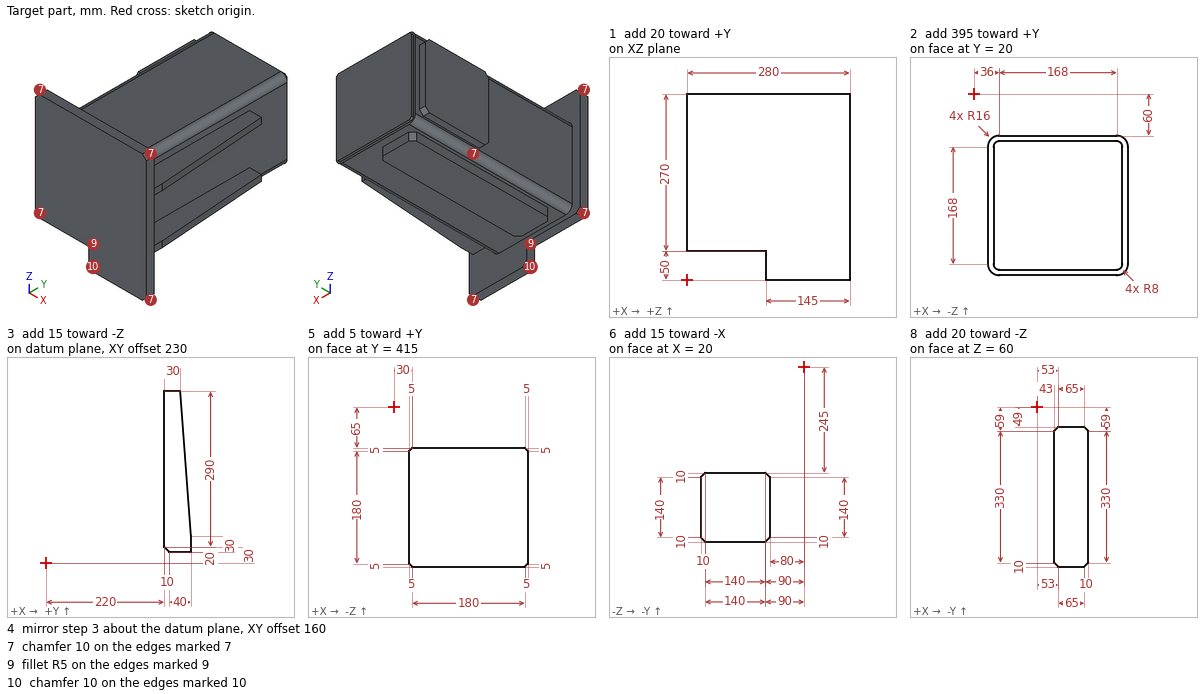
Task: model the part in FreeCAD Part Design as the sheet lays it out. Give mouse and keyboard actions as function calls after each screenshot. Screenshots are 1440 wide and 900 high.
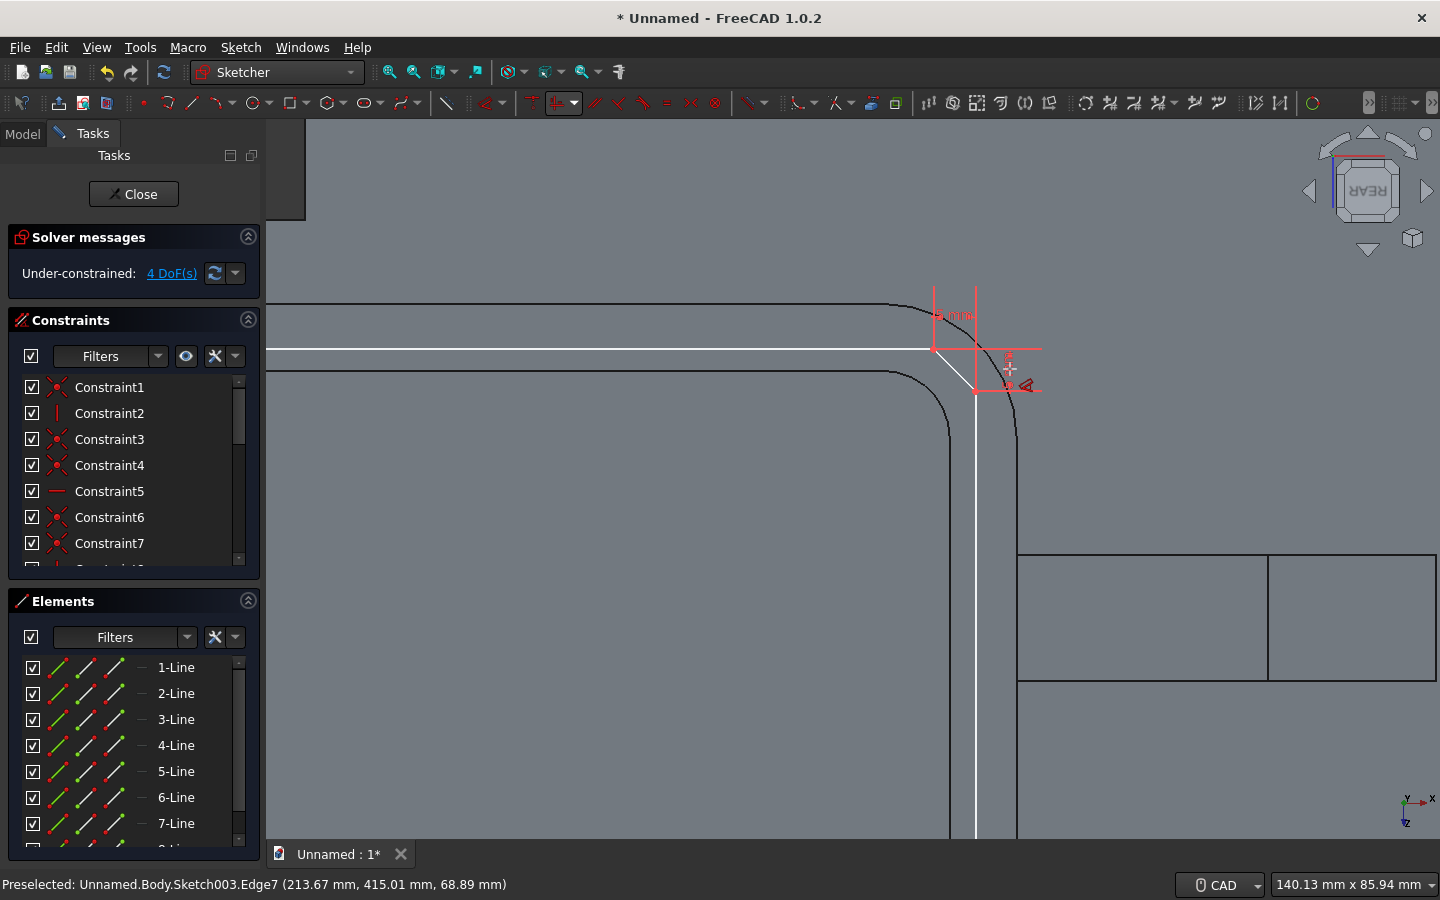
scroll(964, 380, down, 8)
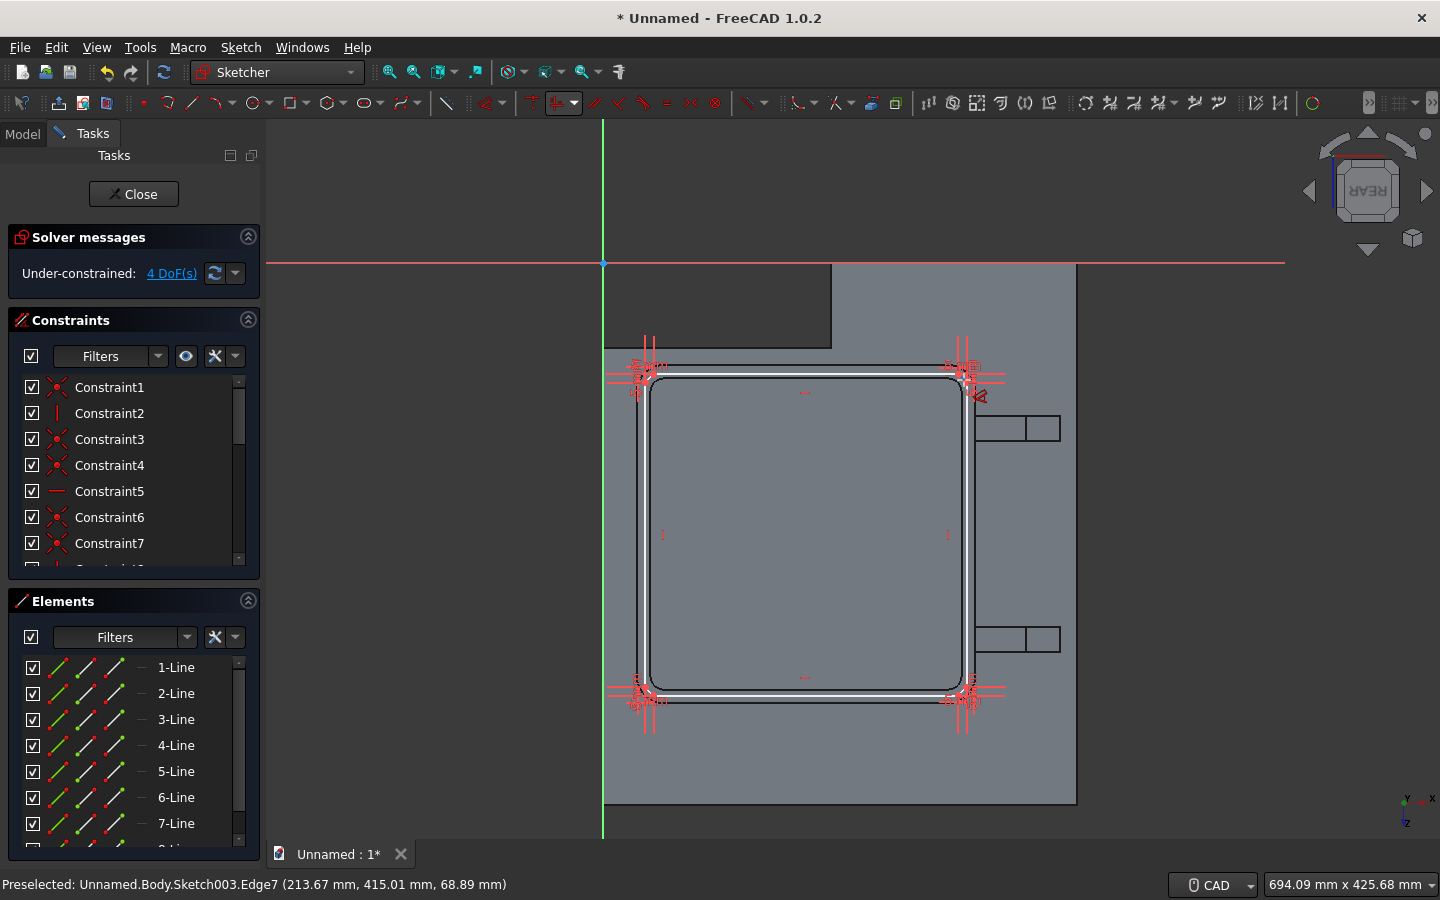
click(645, 474)
click(679, 535)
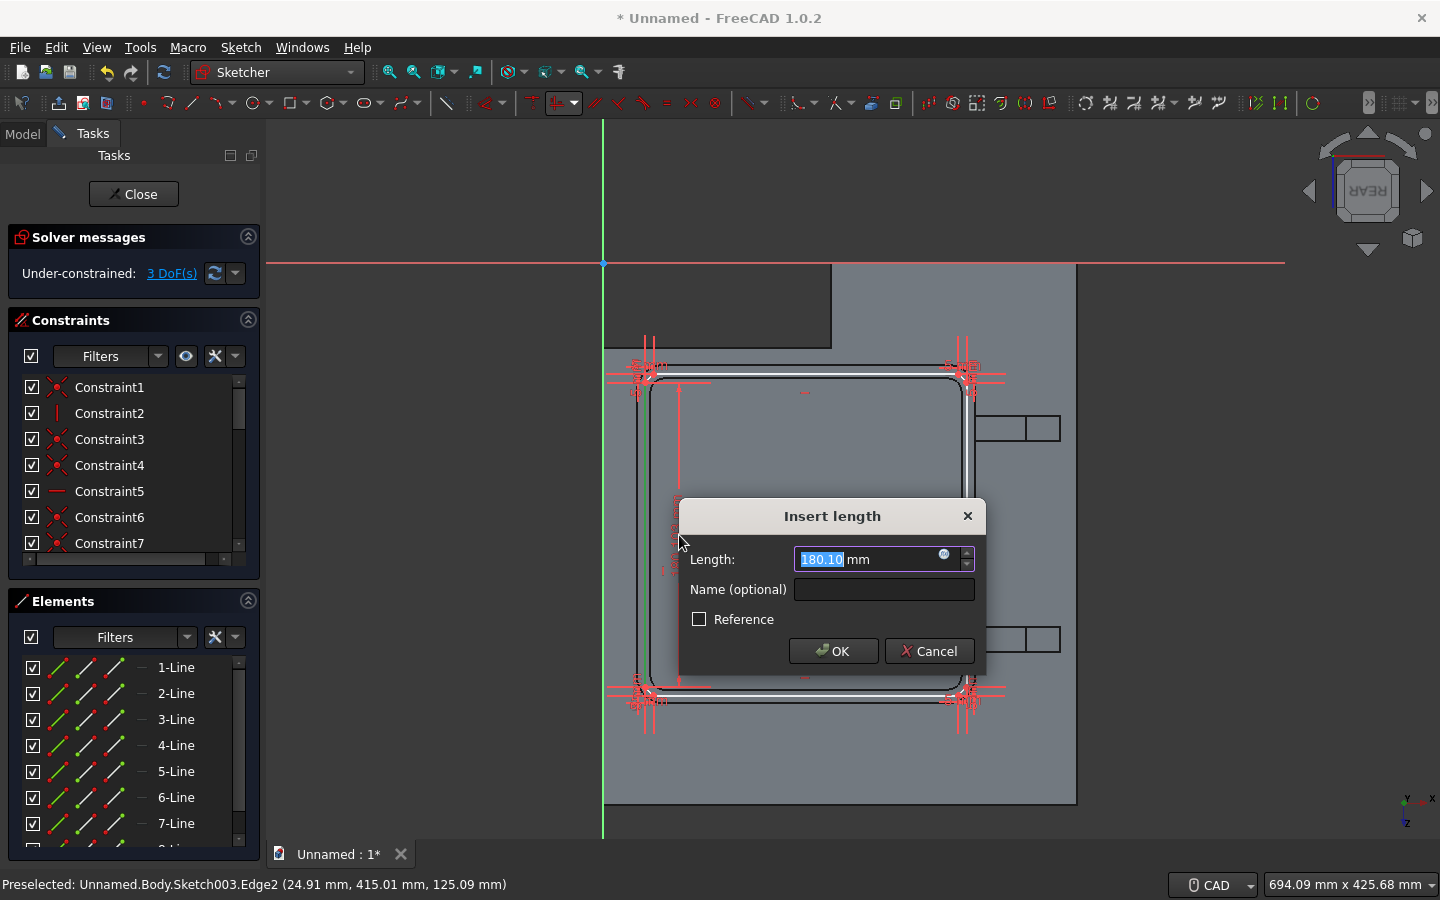
text(180)
key(Return)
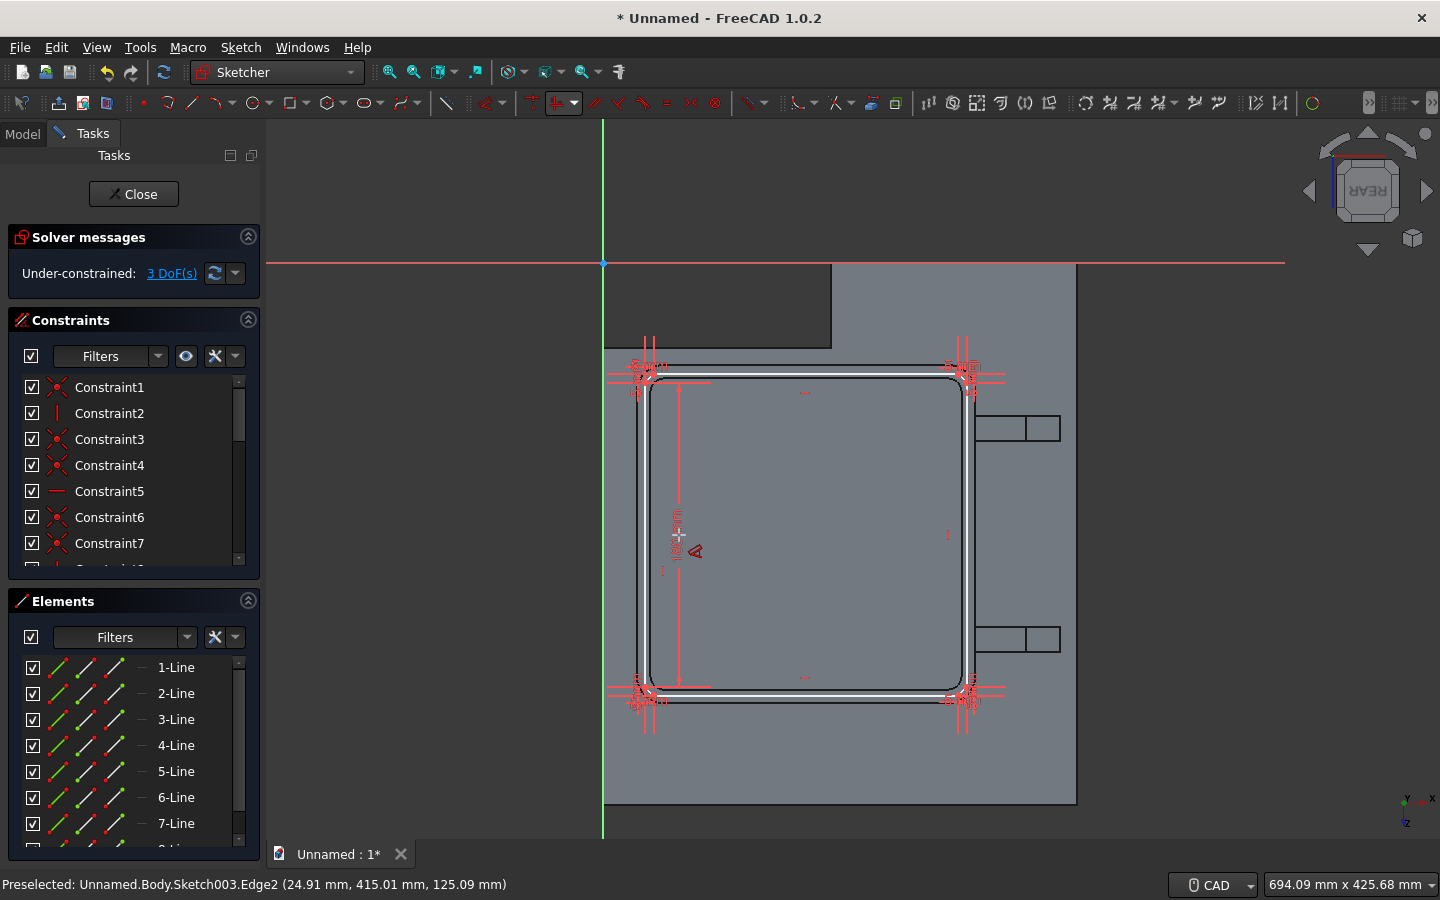
click(745, 696)
click(806, 730)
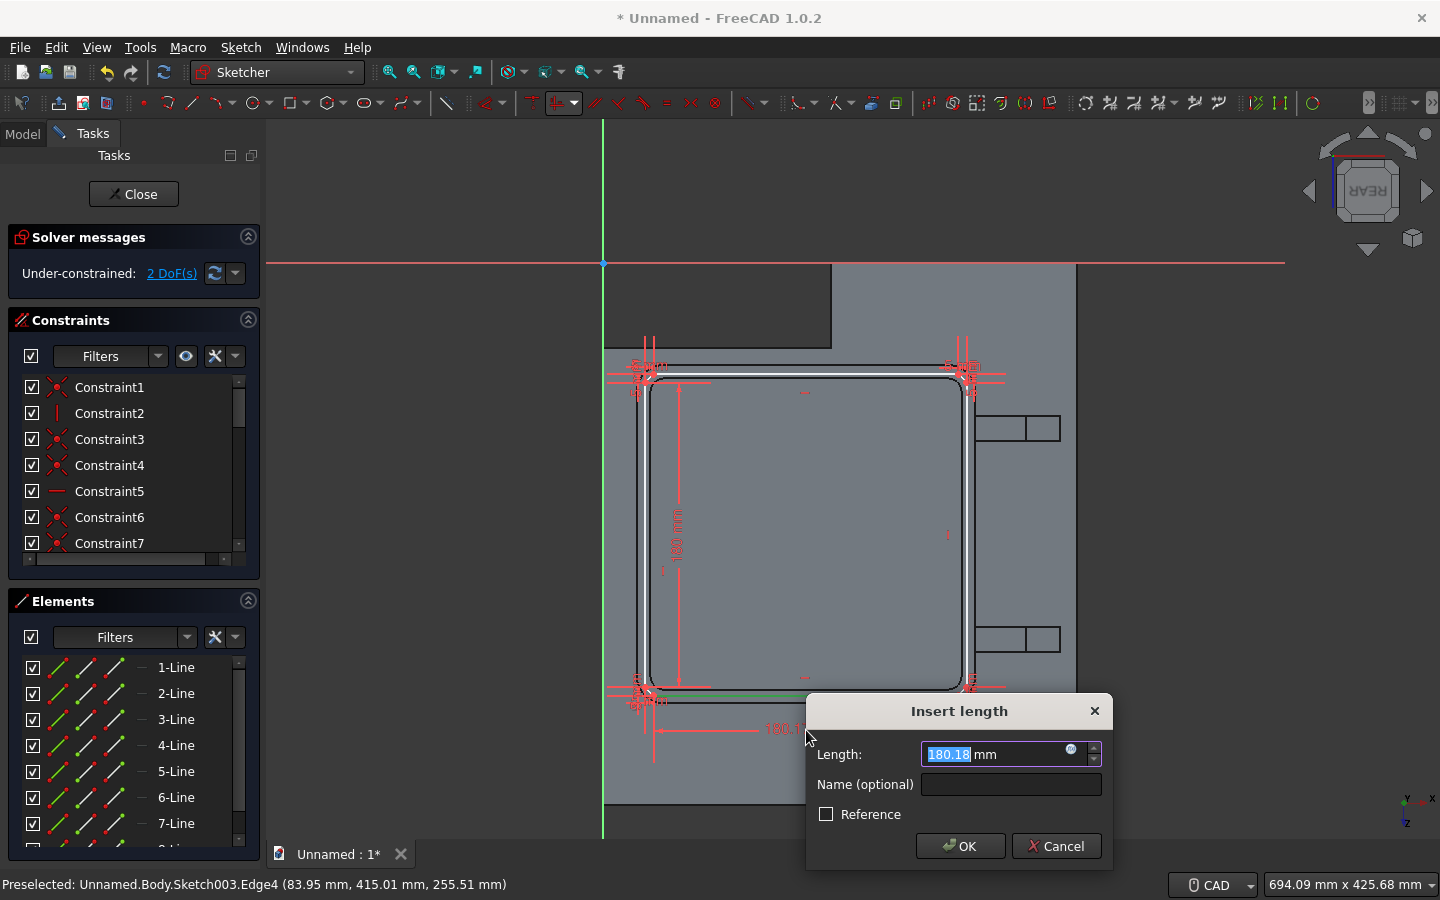
text(180)
key(Return)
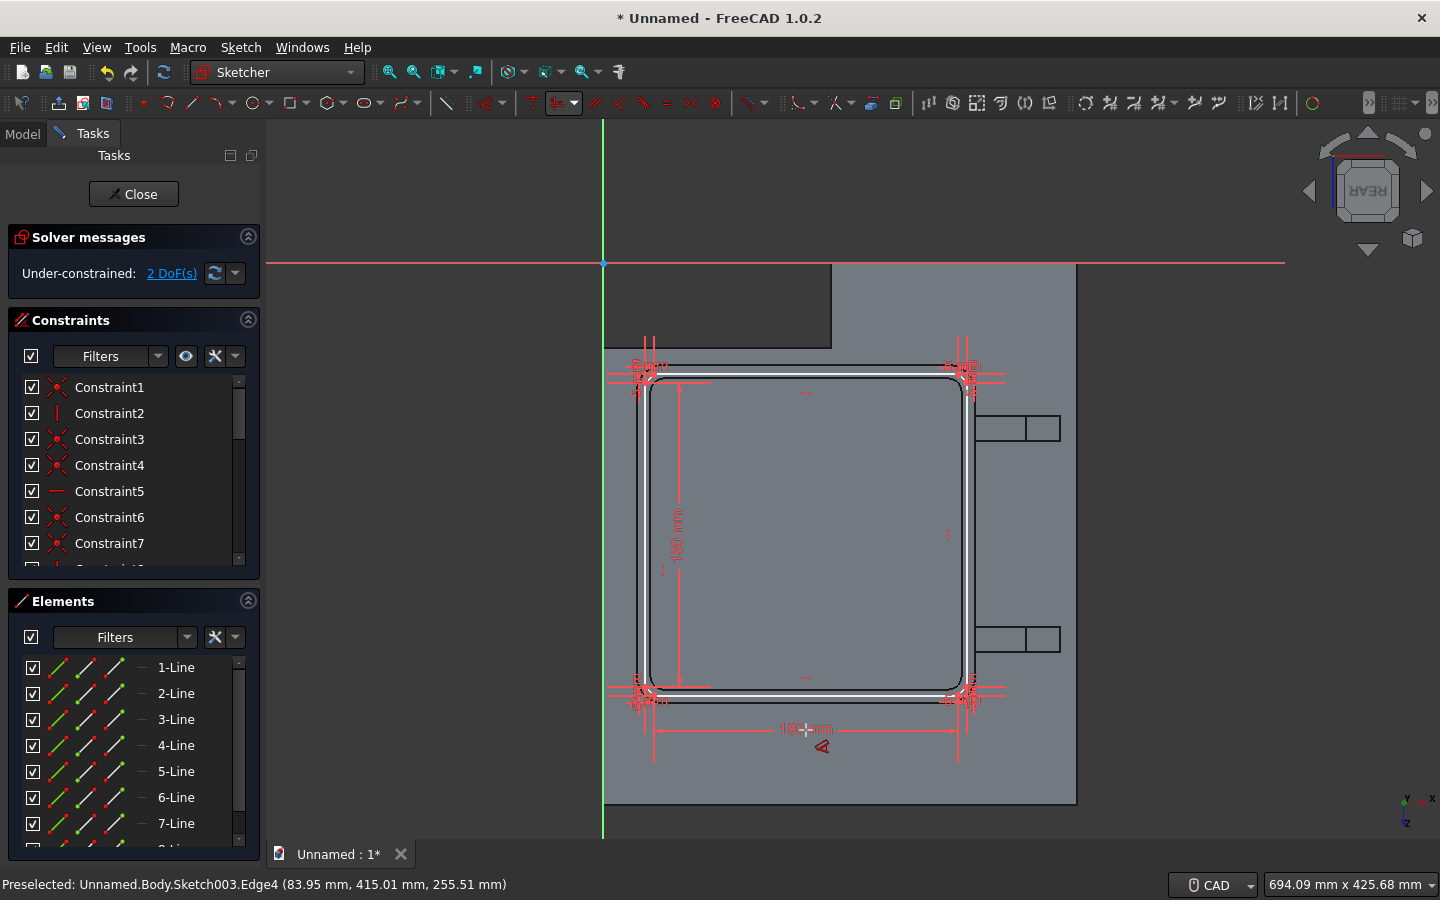
click(654, 374)
click(628, 229)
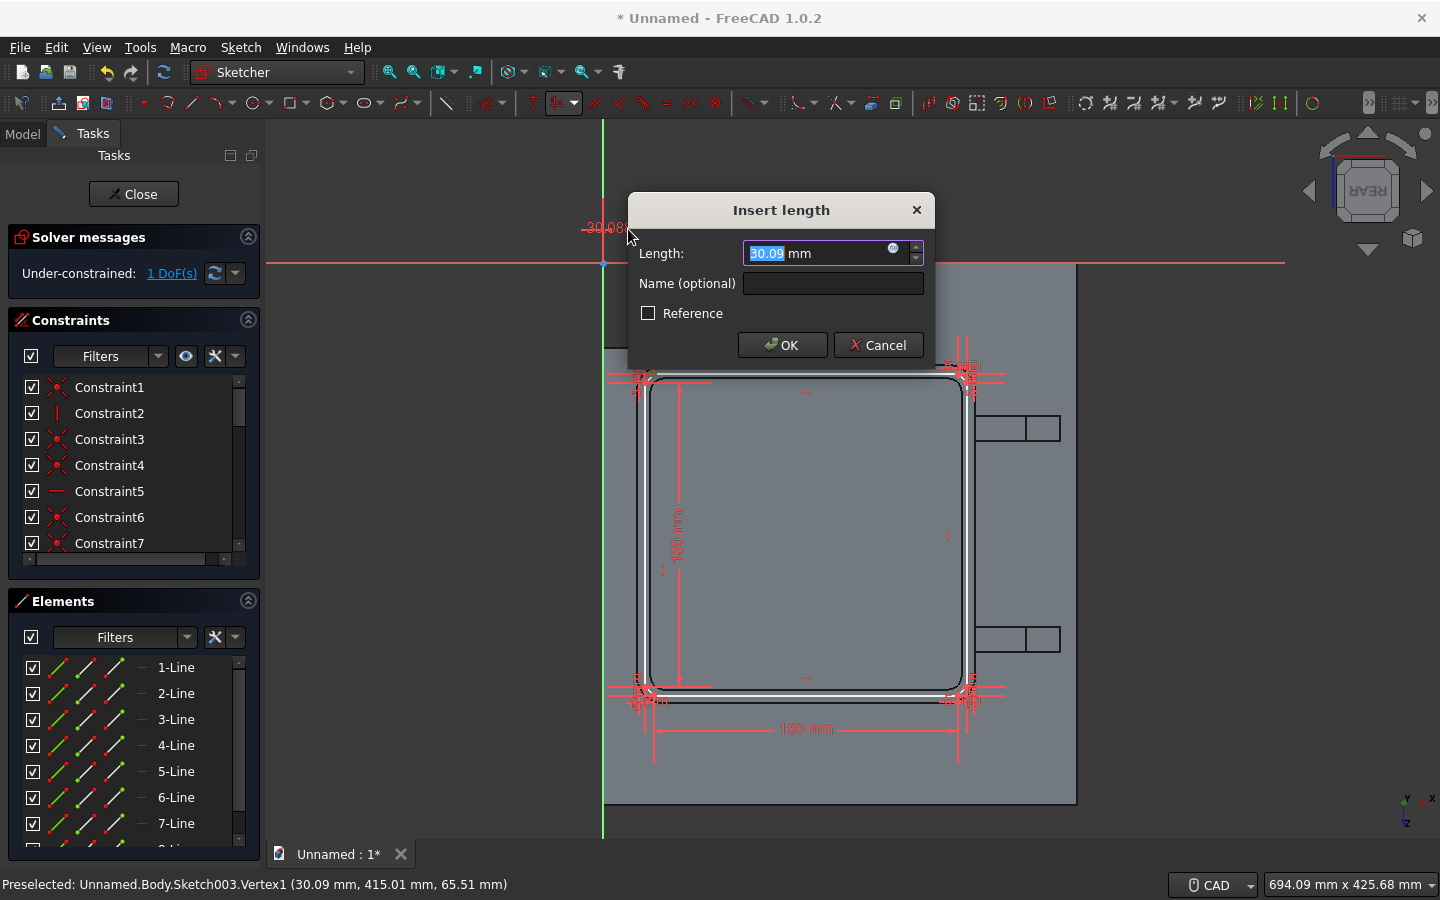
text(30)
key(Return)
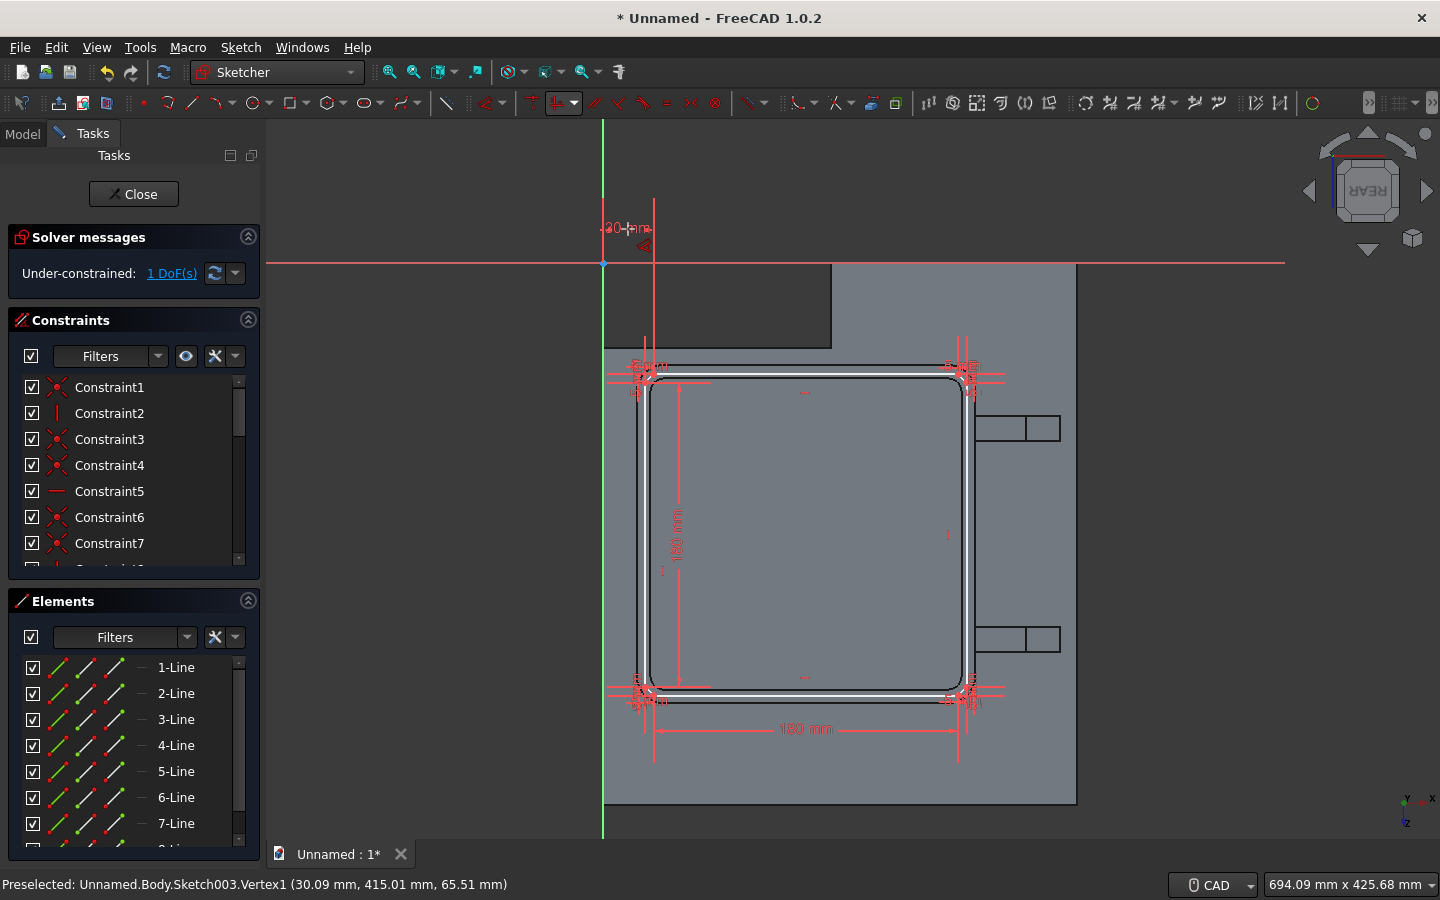
click(654, 374)
click(569, 319)